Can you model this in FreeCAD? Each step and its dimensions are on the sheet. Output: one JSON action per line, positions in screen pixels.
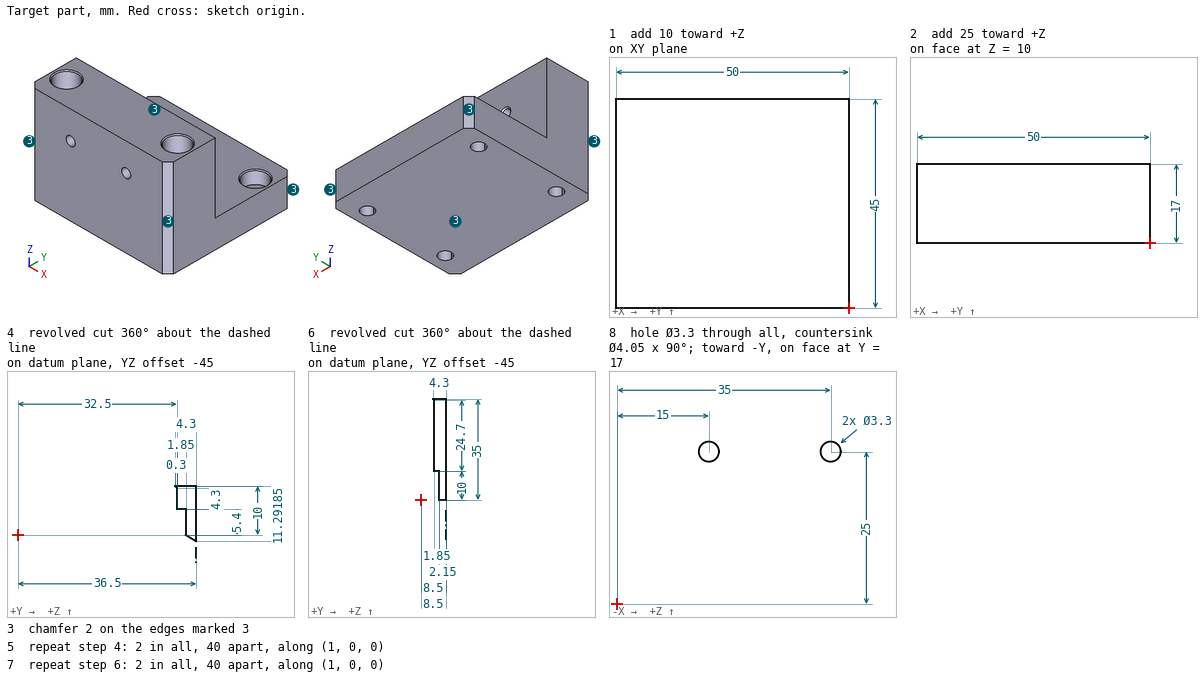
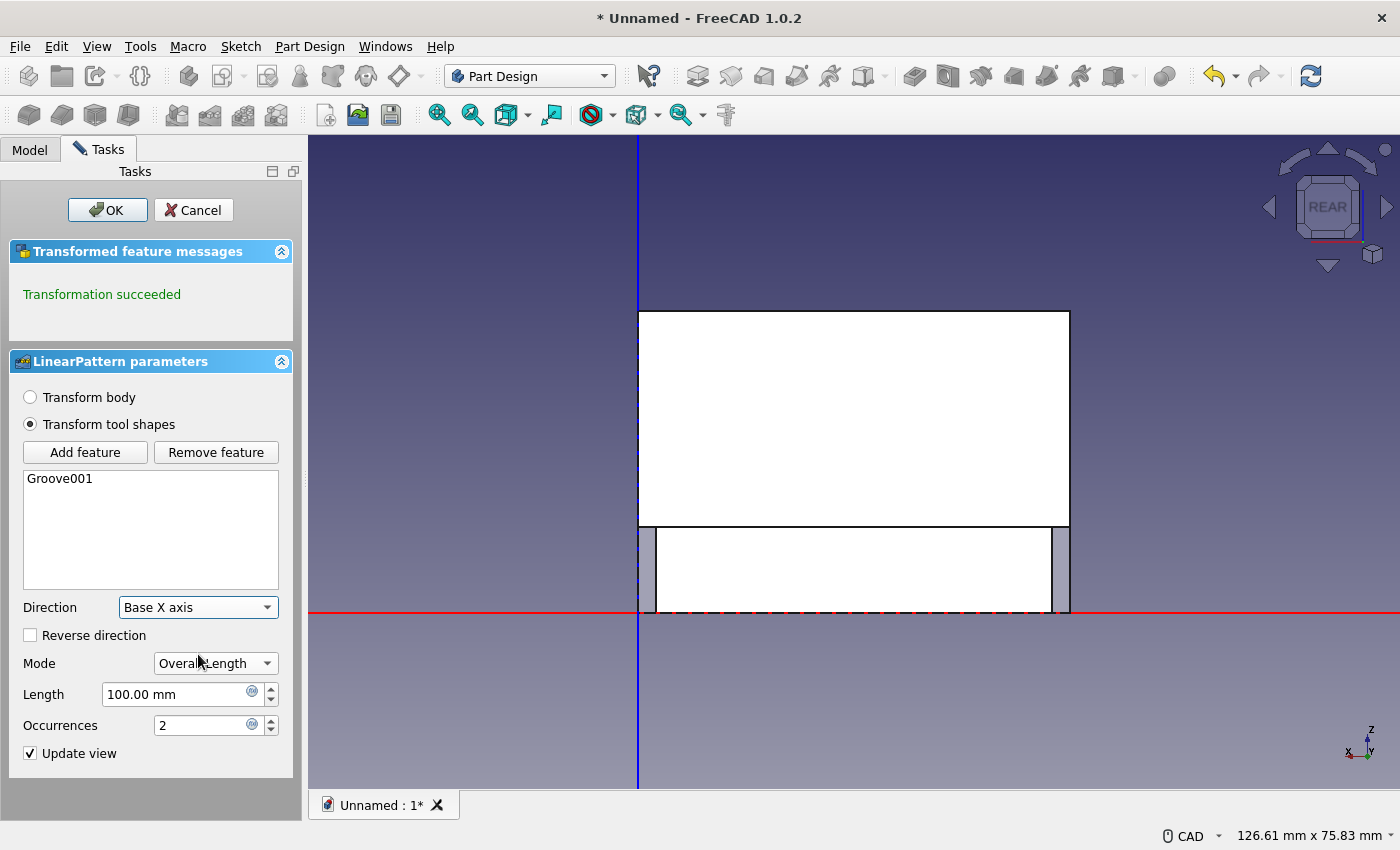
{"action": "left_click", "coordinate": [216, 664]}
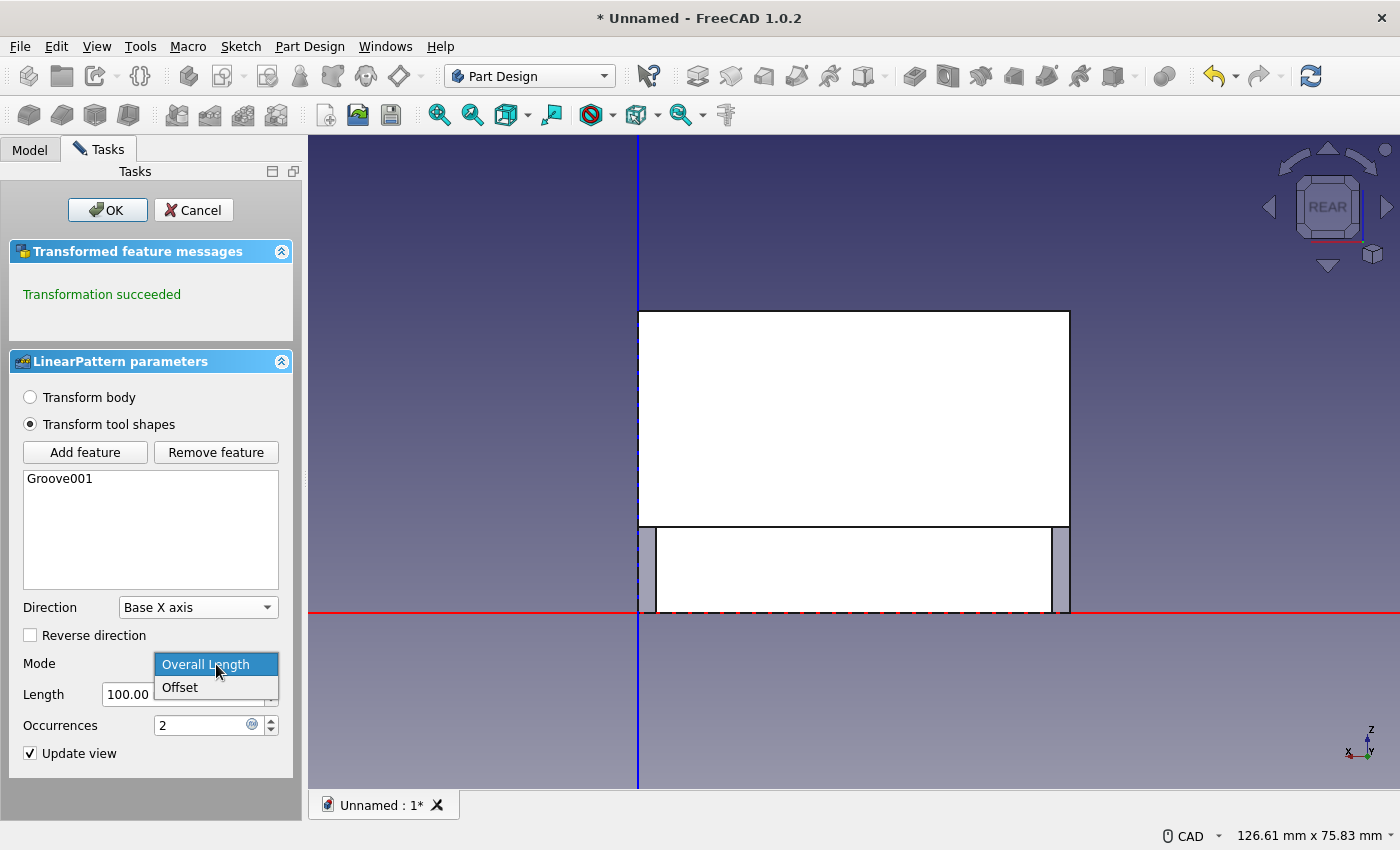
{"action": "left_click", "coordinate": [214, 688]}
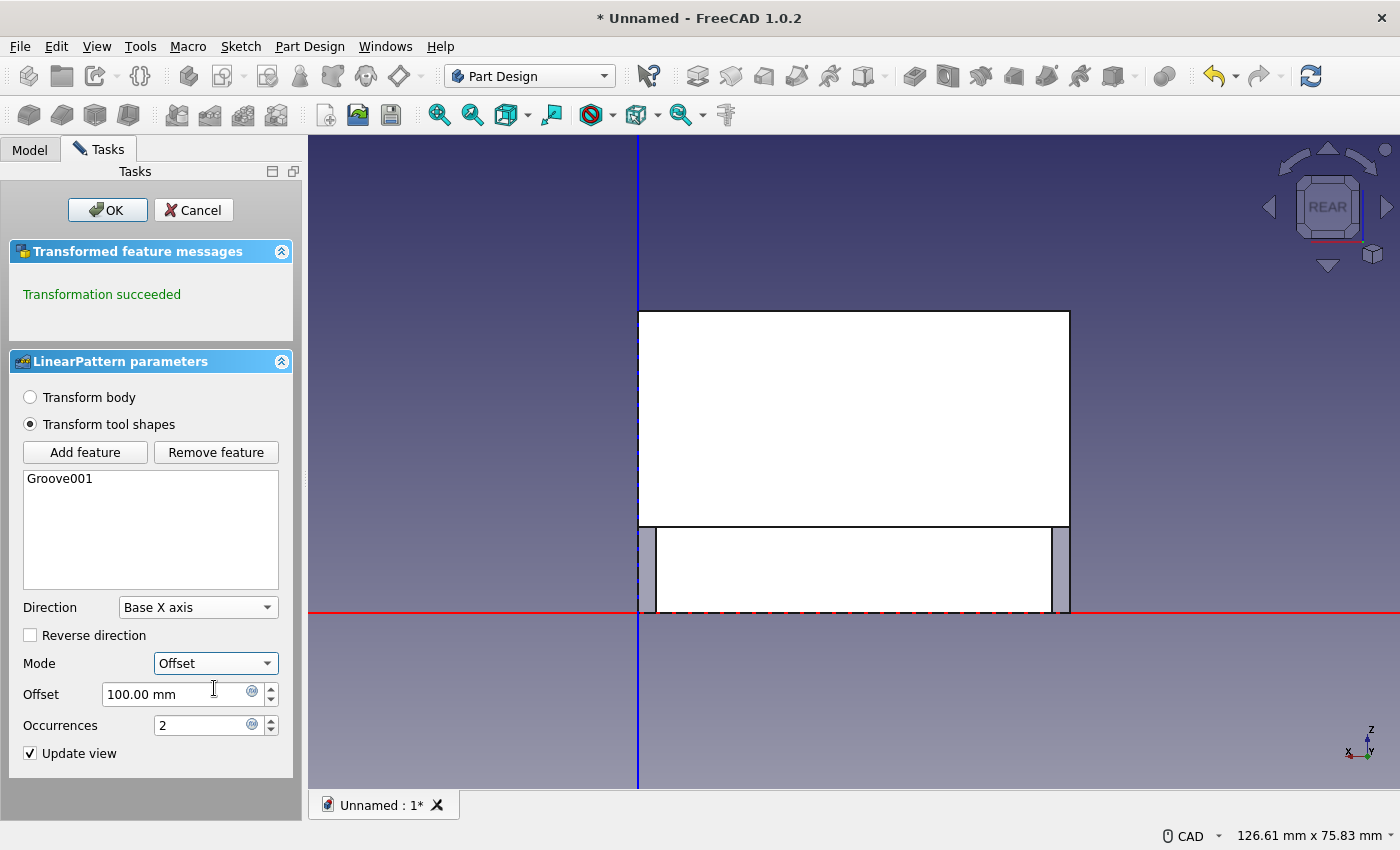
{"action": "triple_click", "coordinate": [184, 694]}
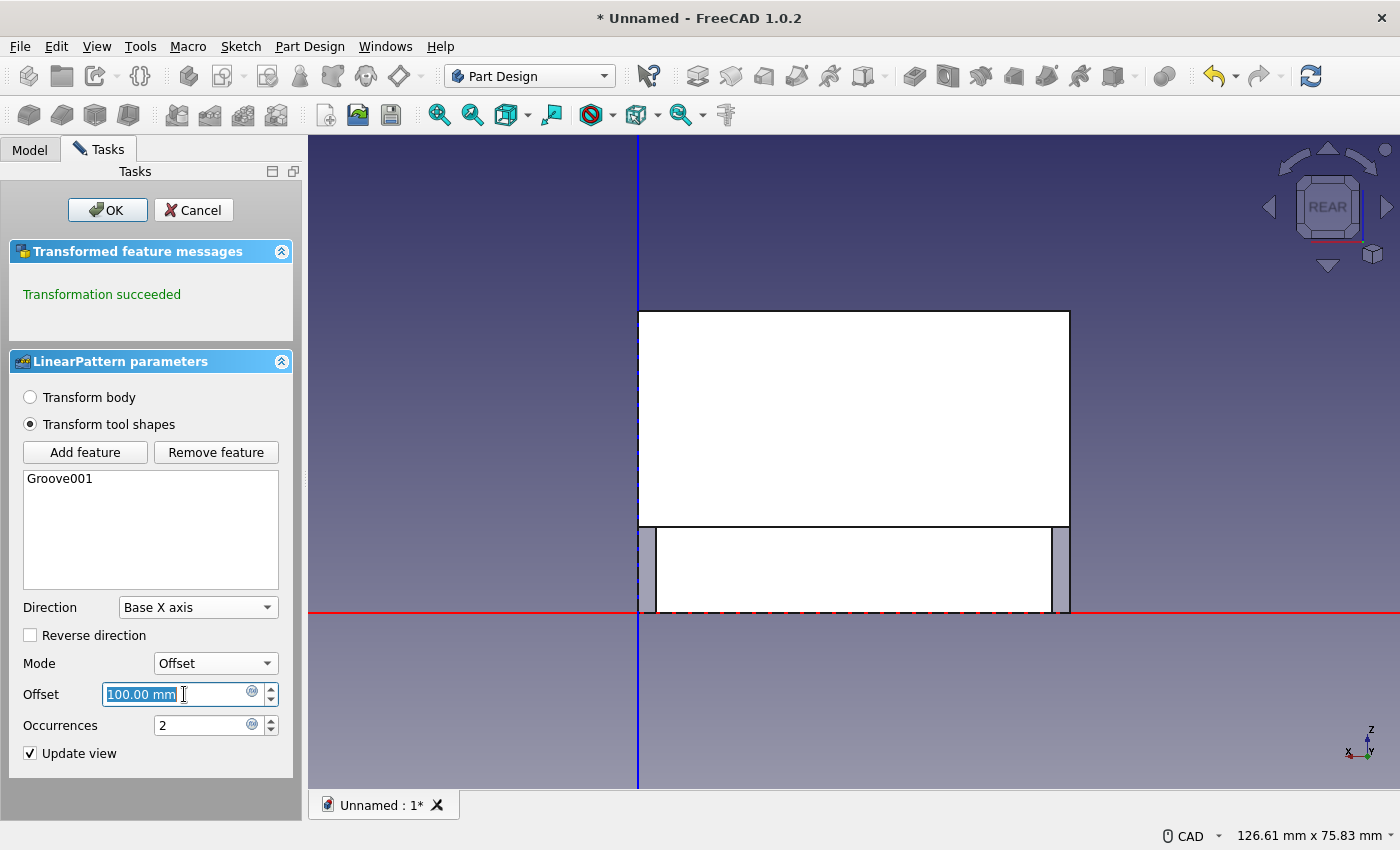
{"action": "type", "text": "40"}
{"action": "key", "text": "Tab"}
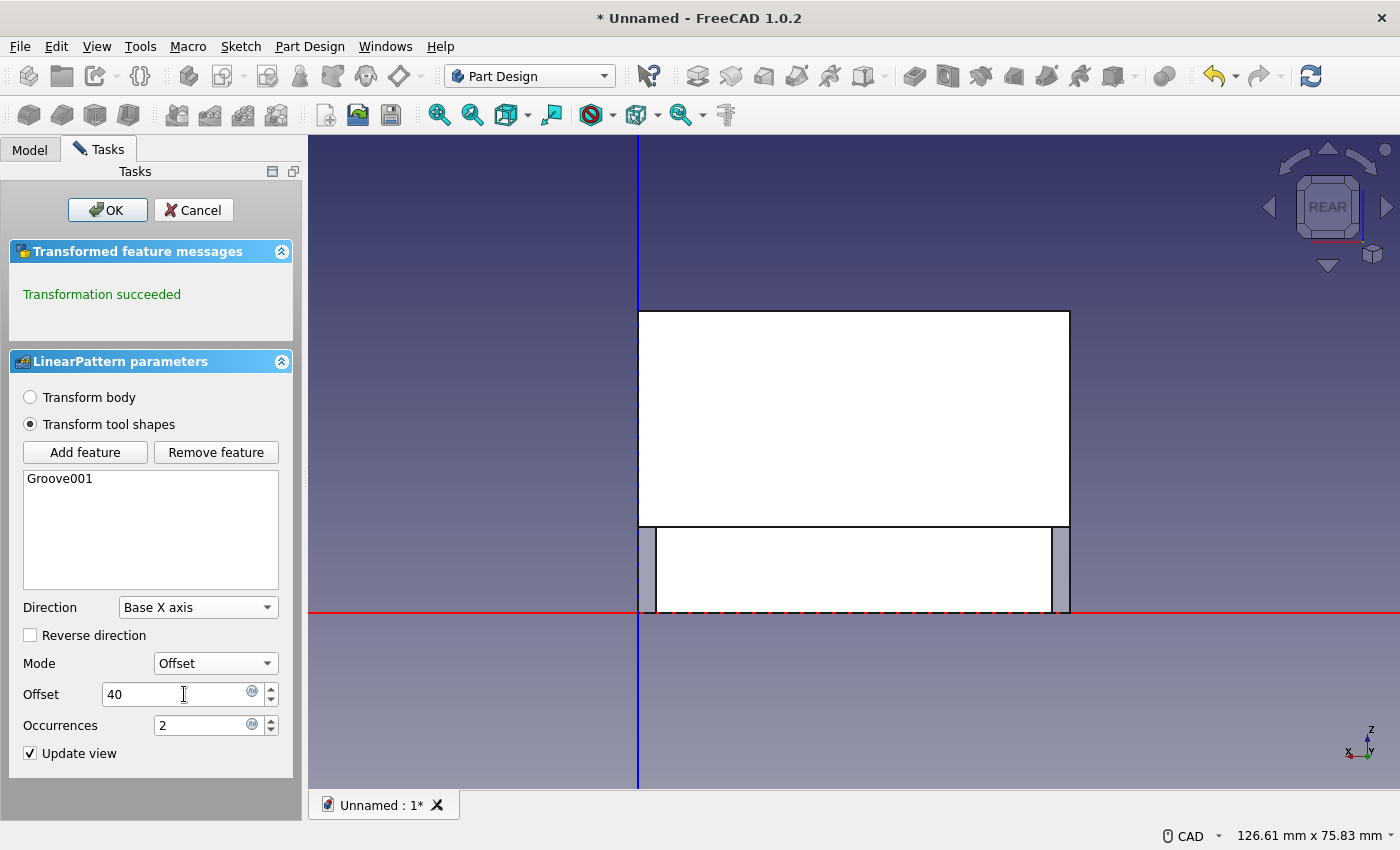
{"action": "triple_click", "coordinate": [210, 726]}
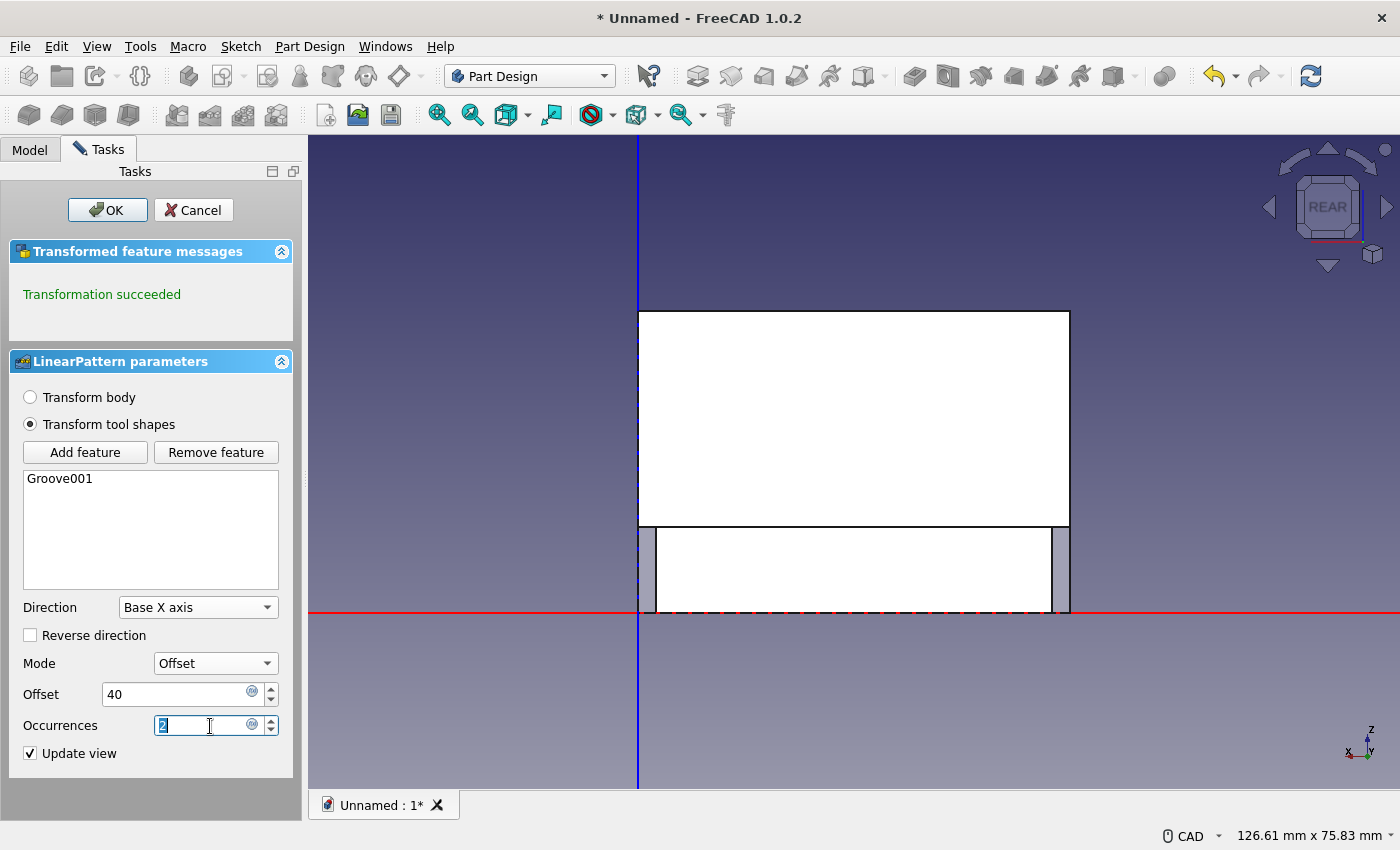
{"action": "type", "text": "2"}
{"action": "key", "text": "Tab"}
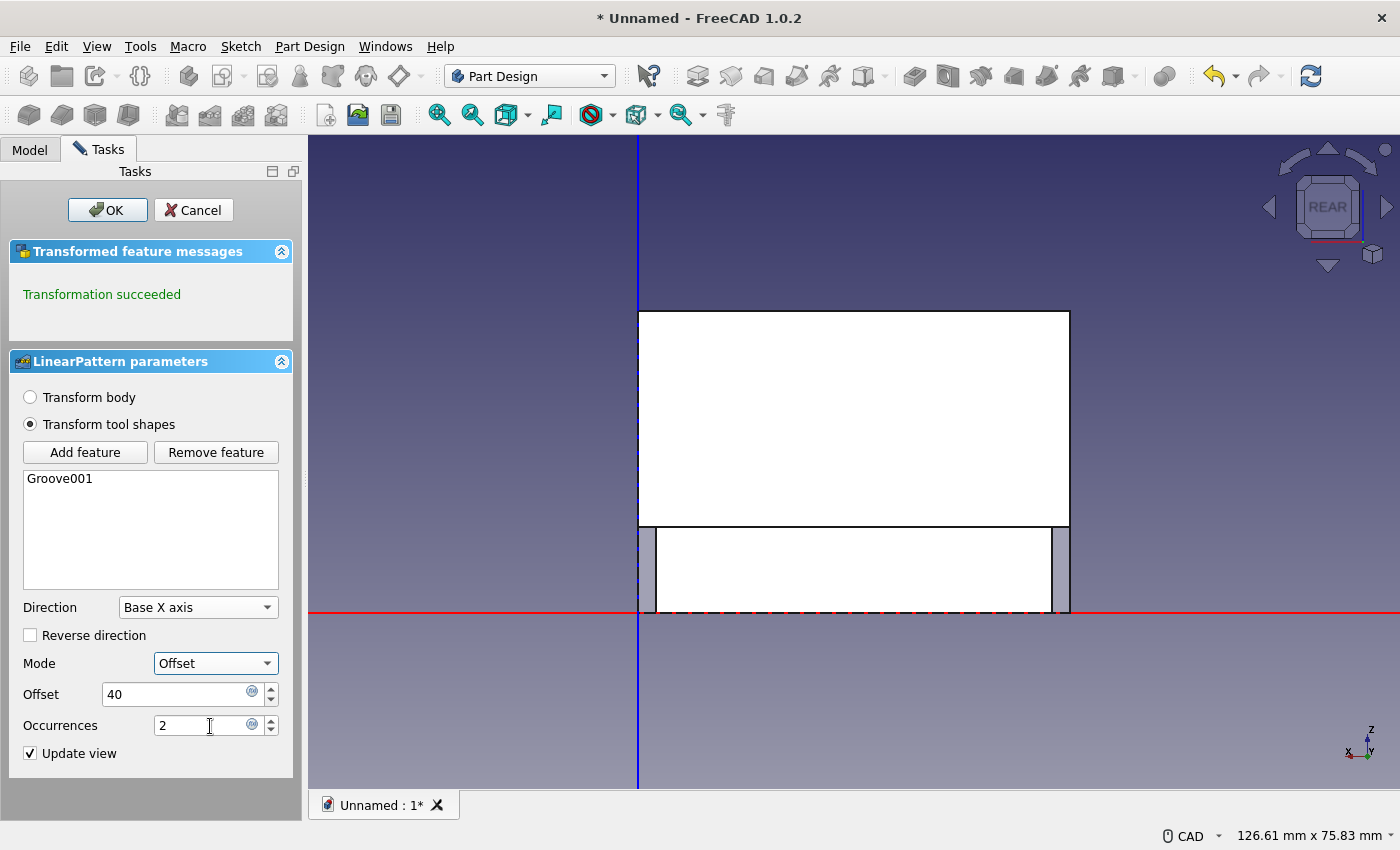
{"action": "left_click", "coordinate": [108, 210]}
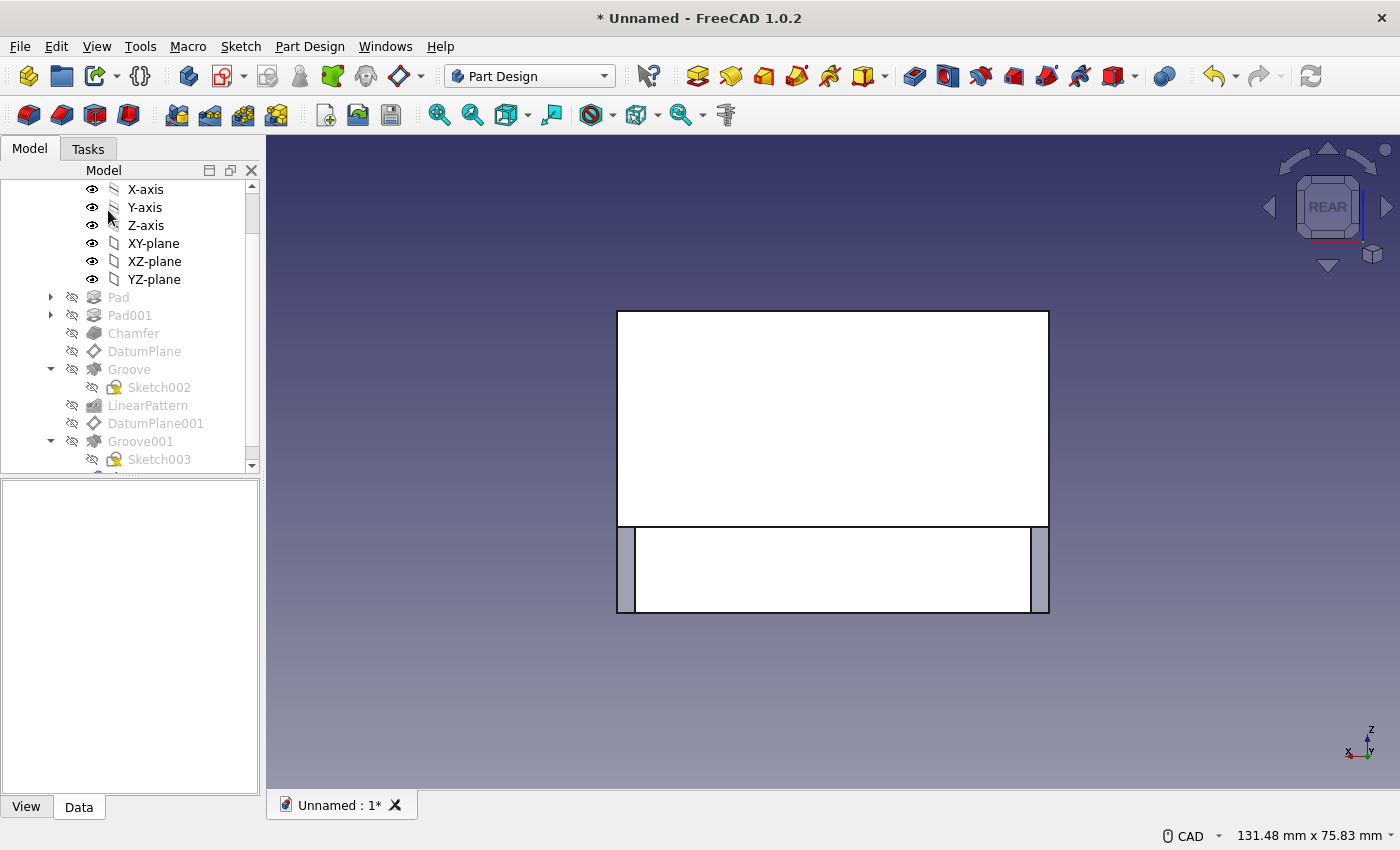
{"action": "left_click", "coordinate": [771, 418]}